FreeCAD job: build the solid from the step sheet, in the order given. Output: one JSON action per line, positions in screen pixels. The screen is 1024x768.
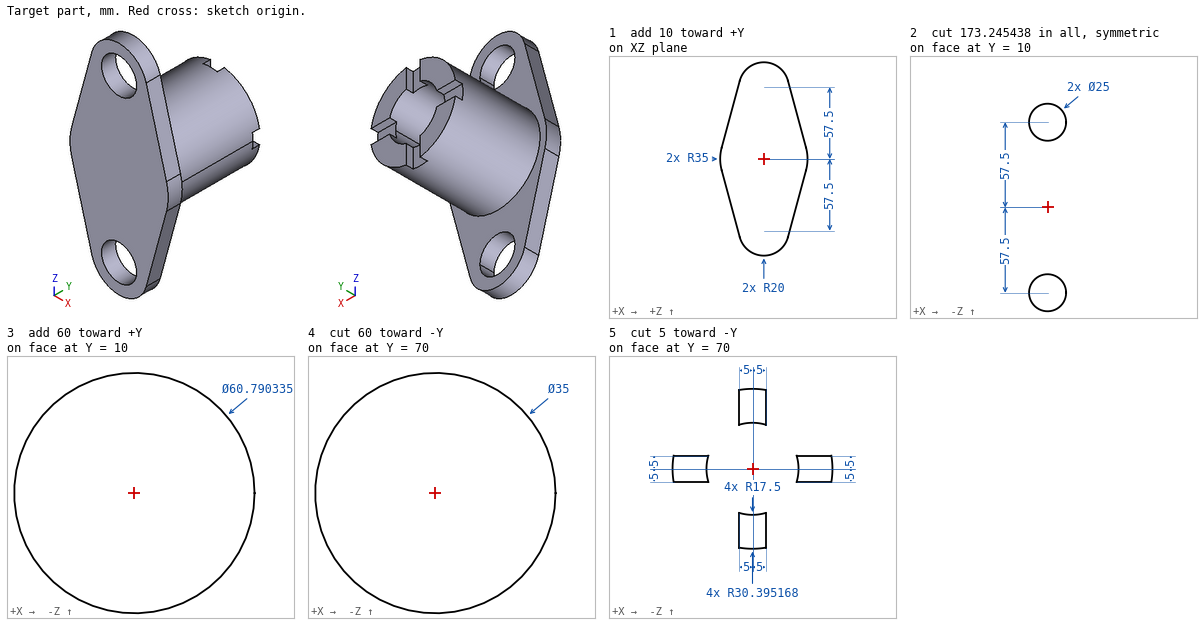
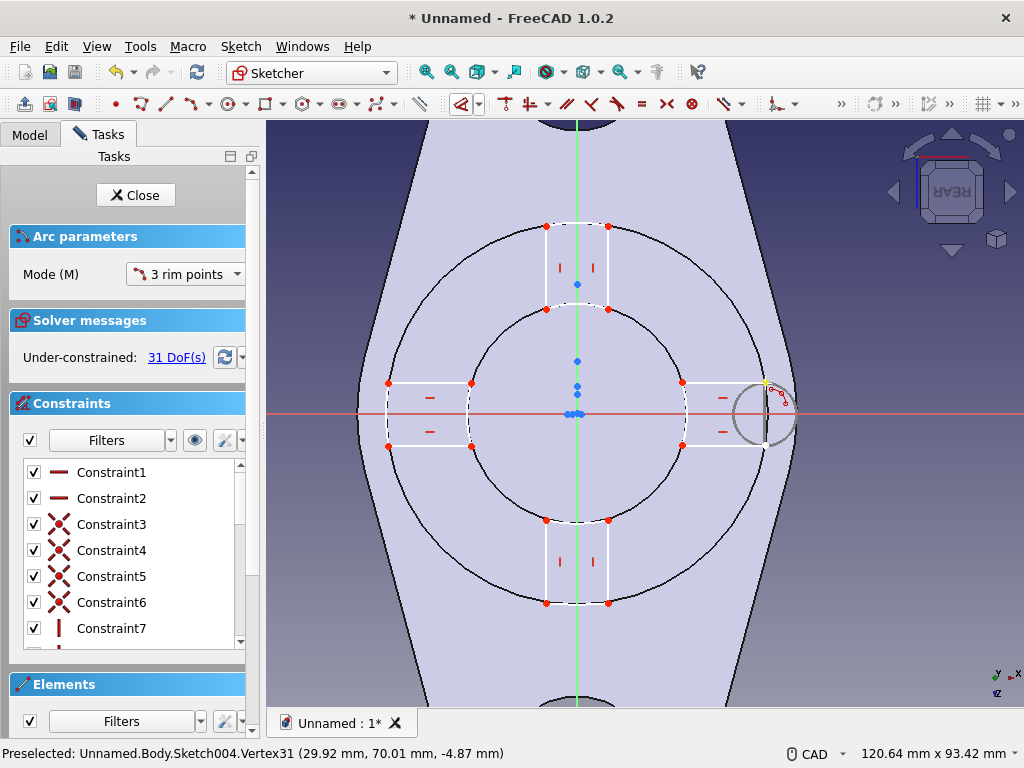
{"action": "scroll", "coordinate": [768, 420], "scroll_direction": "up", "scroll_amount": 10}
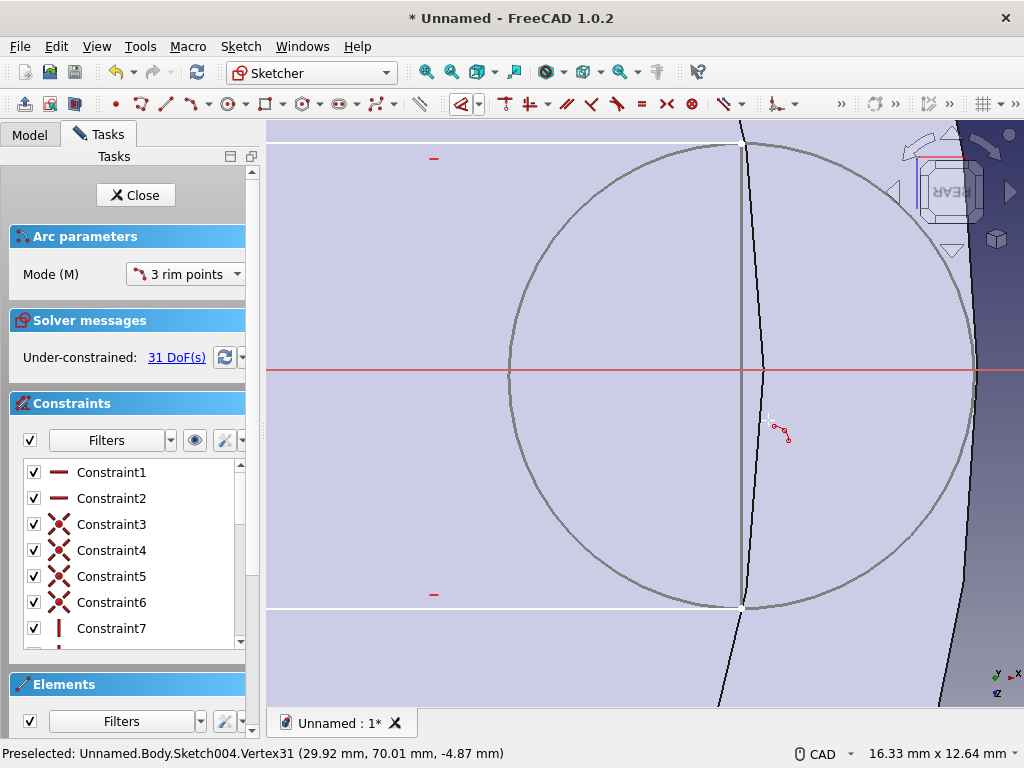
{"action": "left_click", "coordinate": [763, 416]}
{"action": "key", "text": "Escape"}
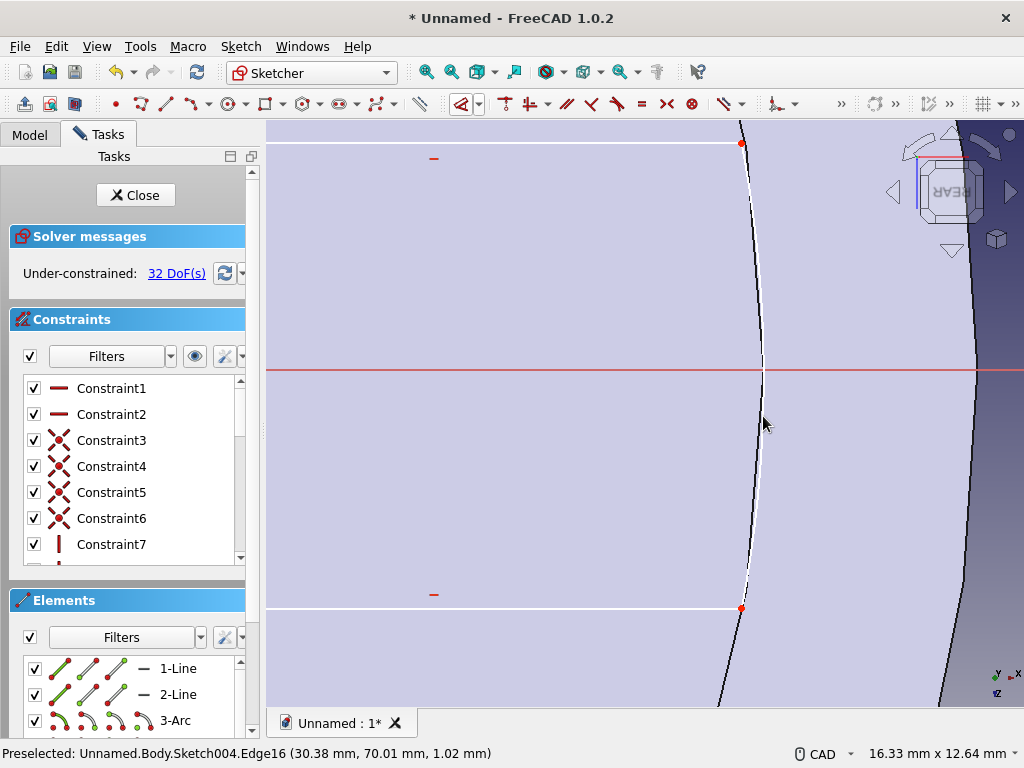
{"action": "scroll", "coordinate": [768, 420], "scroll_direction": "down", "scroll_amount": 10}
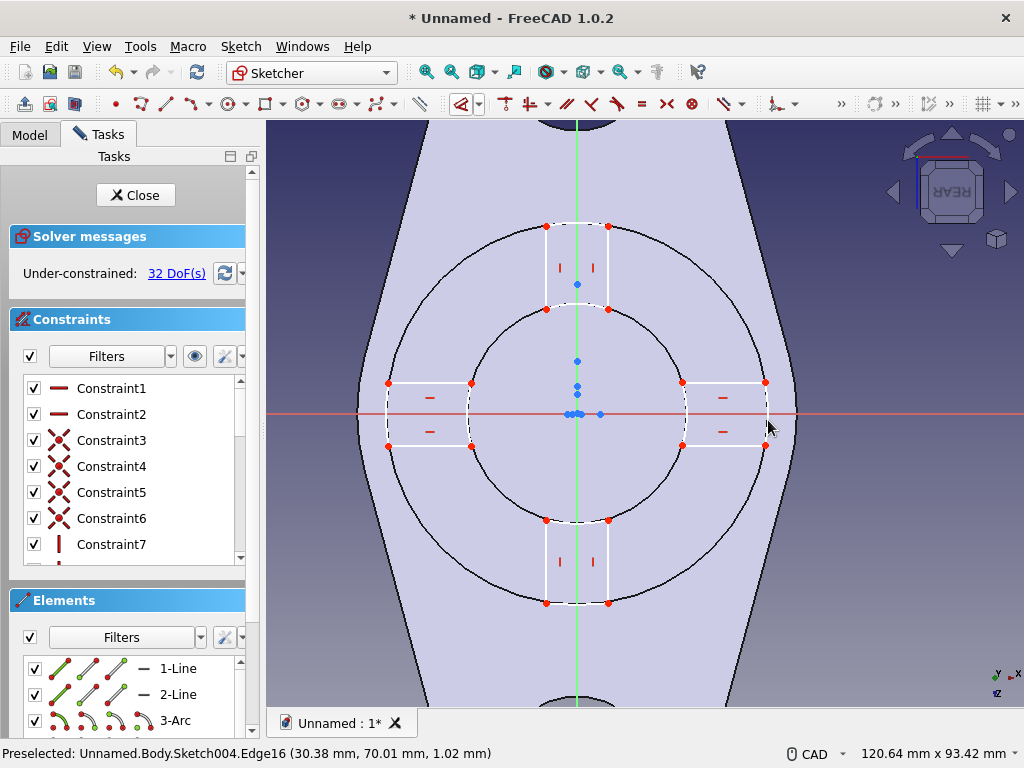
{"action": "left_click", "coordinate": [468, 402]}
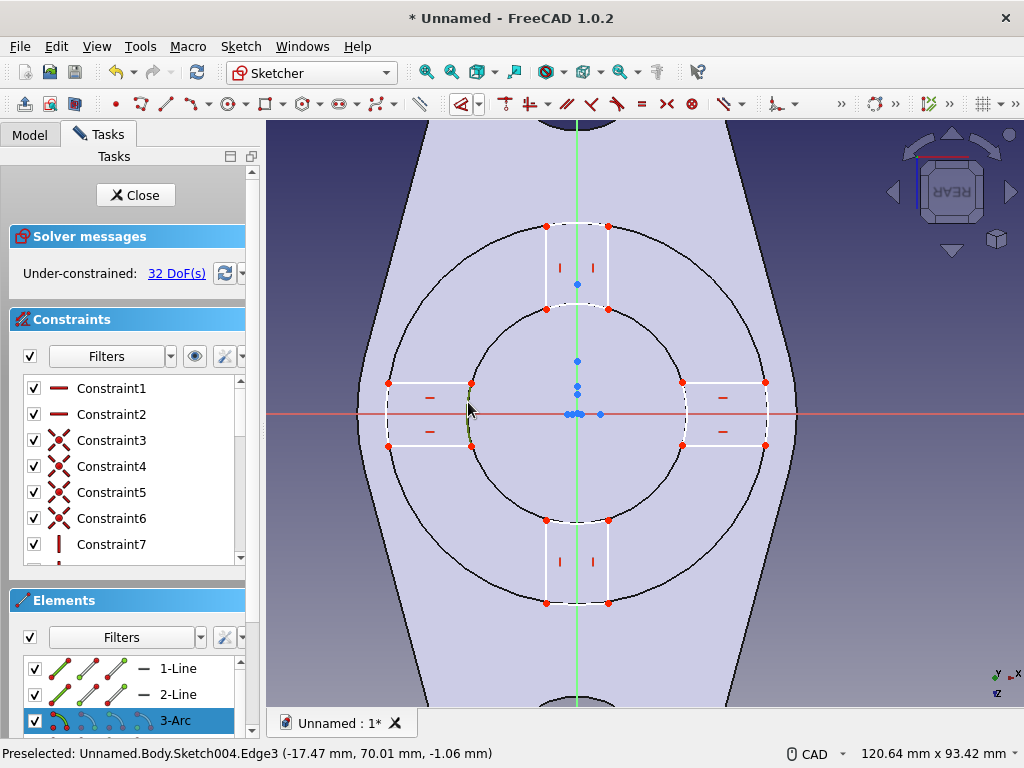
{"action": "left_click", "coordinate": [386, 402]}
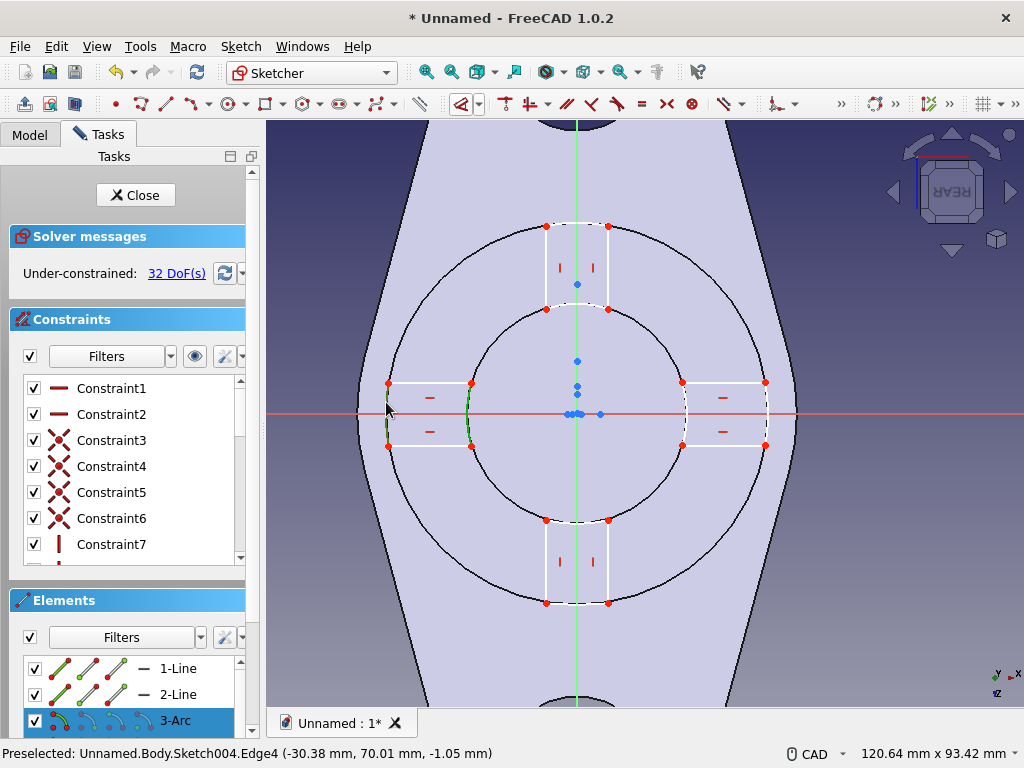
{"action": "key", "text": "c"}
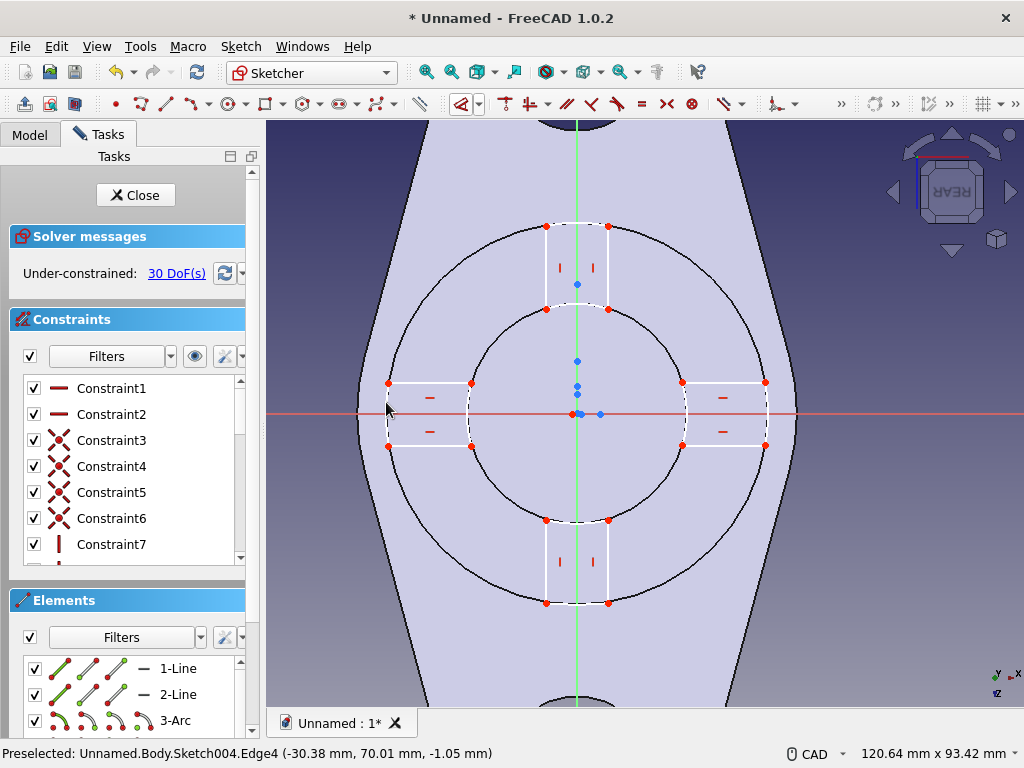
{"action": "left_click", "coordinate": [468, 402]}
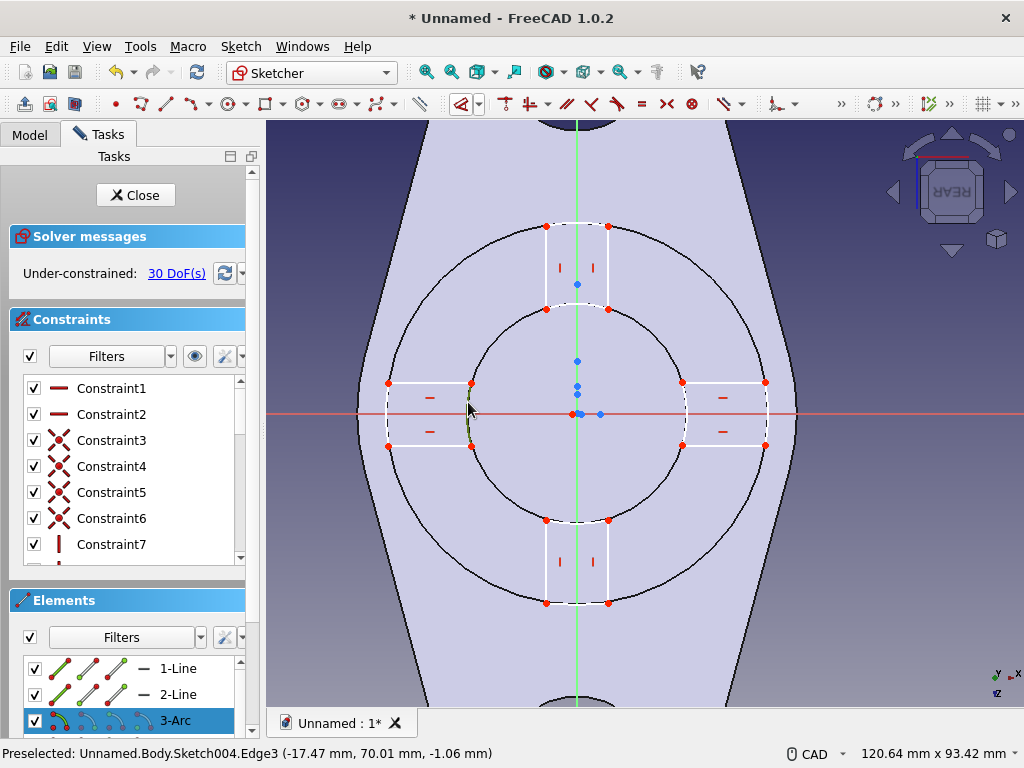
{"action": "left_click", "coordinate": [565, 604]}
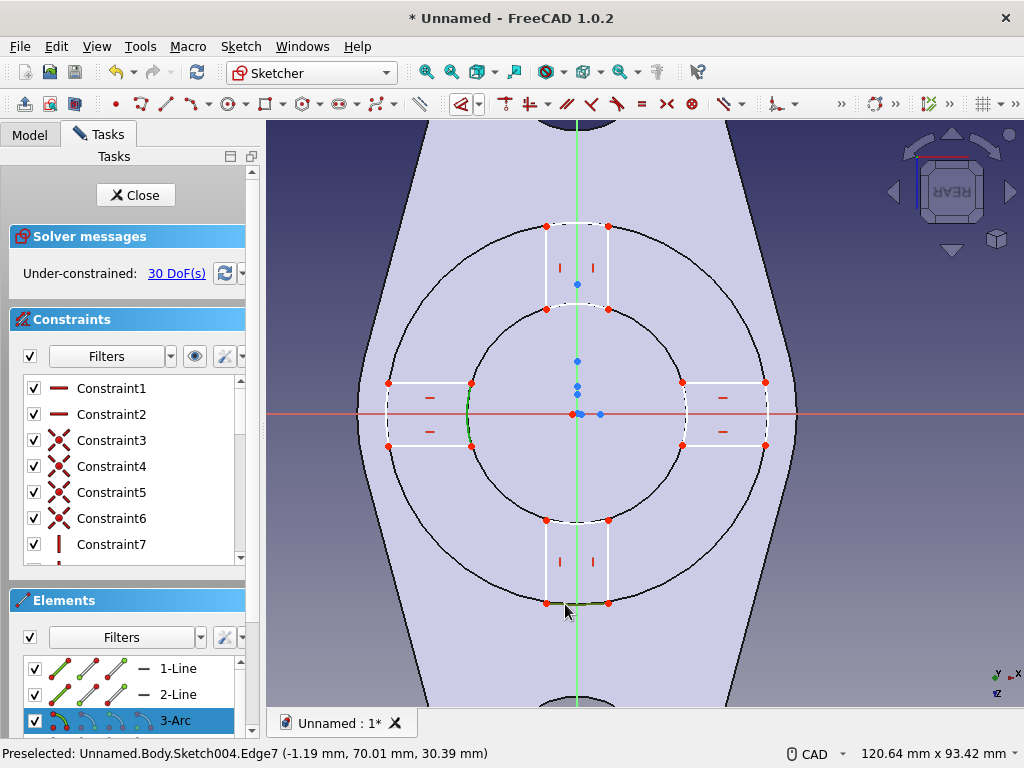
{"action": "left_click", "coordinate": [505, 104]}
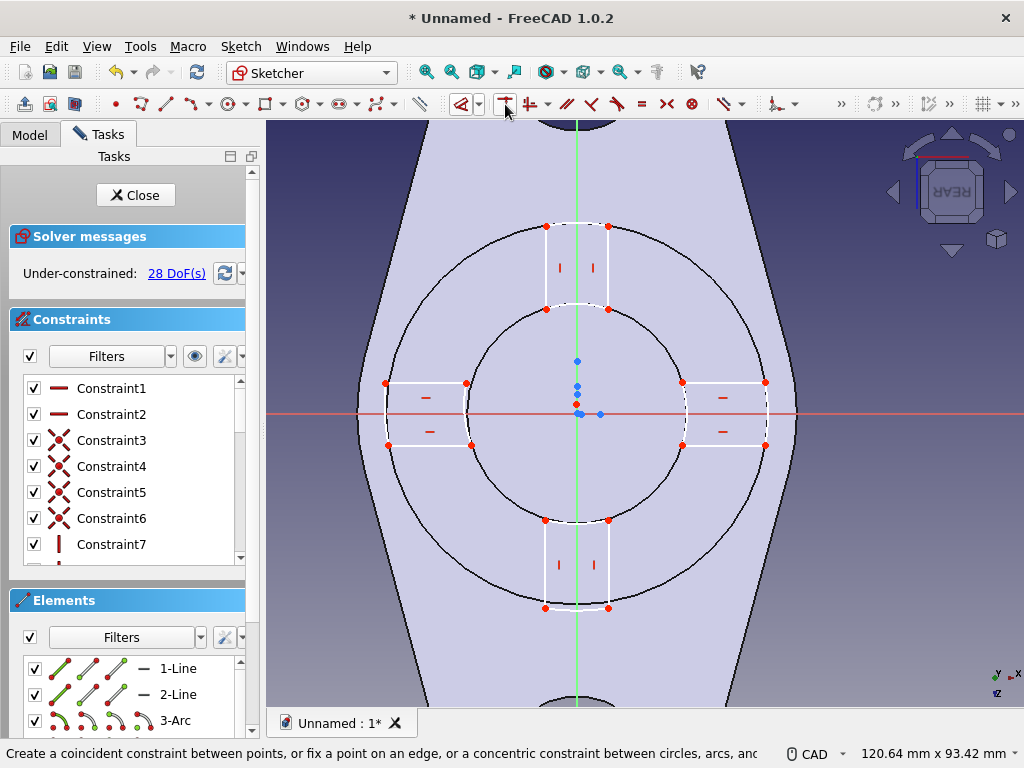
{"action": "left_click", "coordinate": [464, 402]}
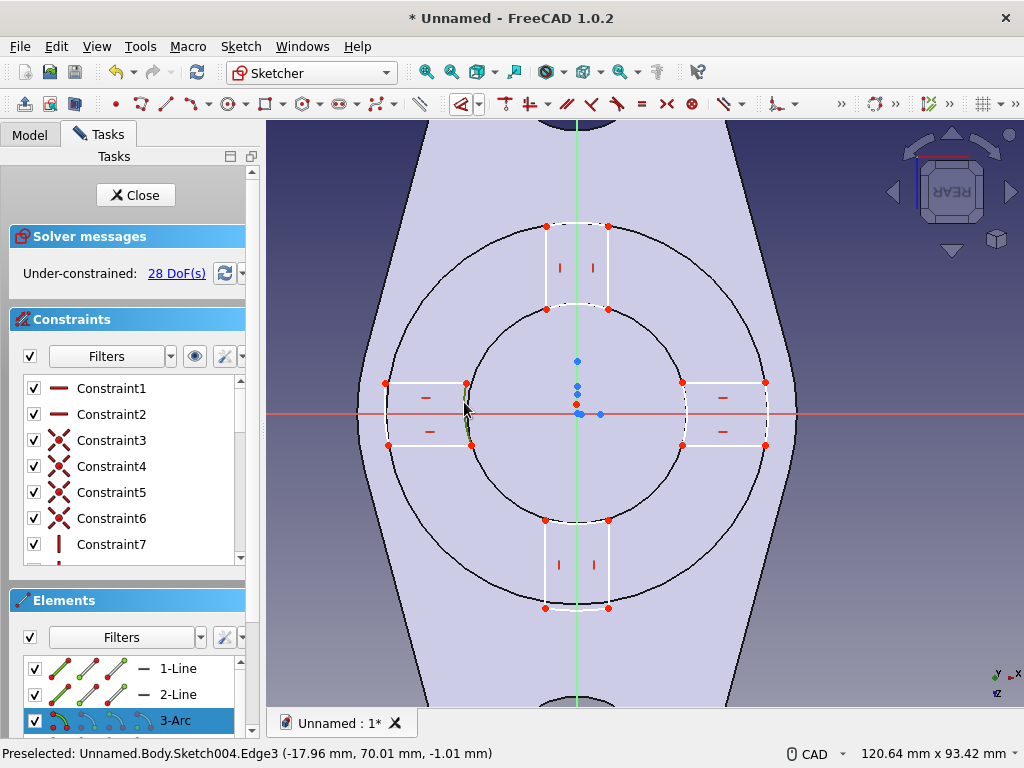
{"action": "left_click", "coordinate": [564, 523]}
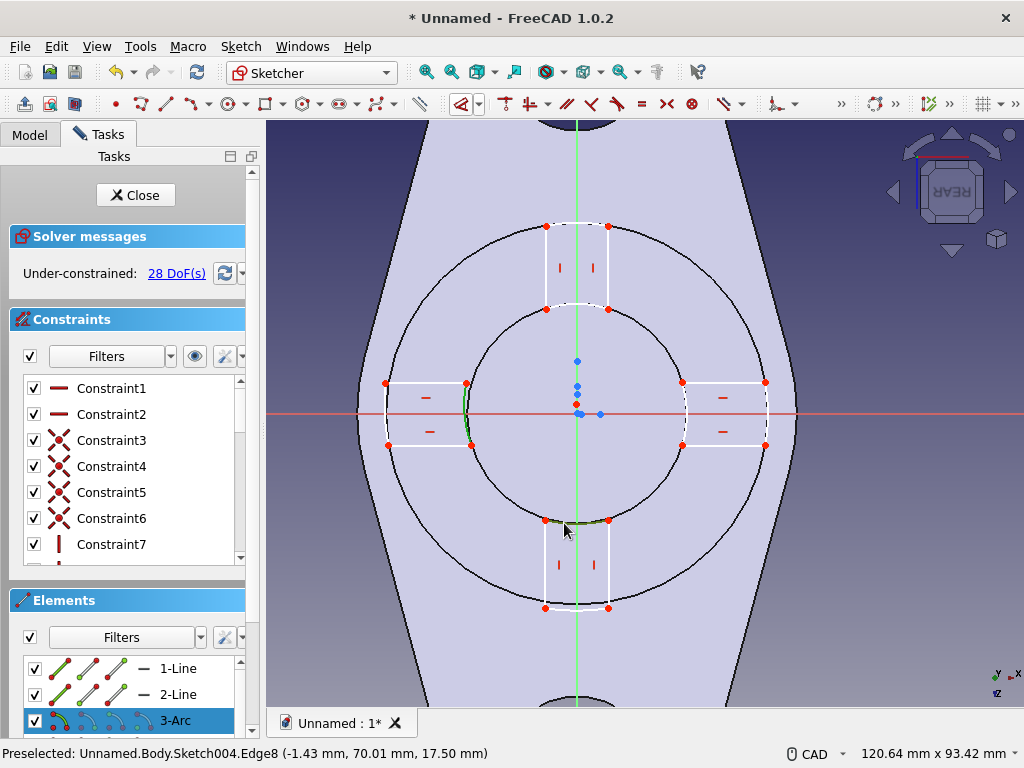
{"action": "left_click", "coordinate": [505, 104]}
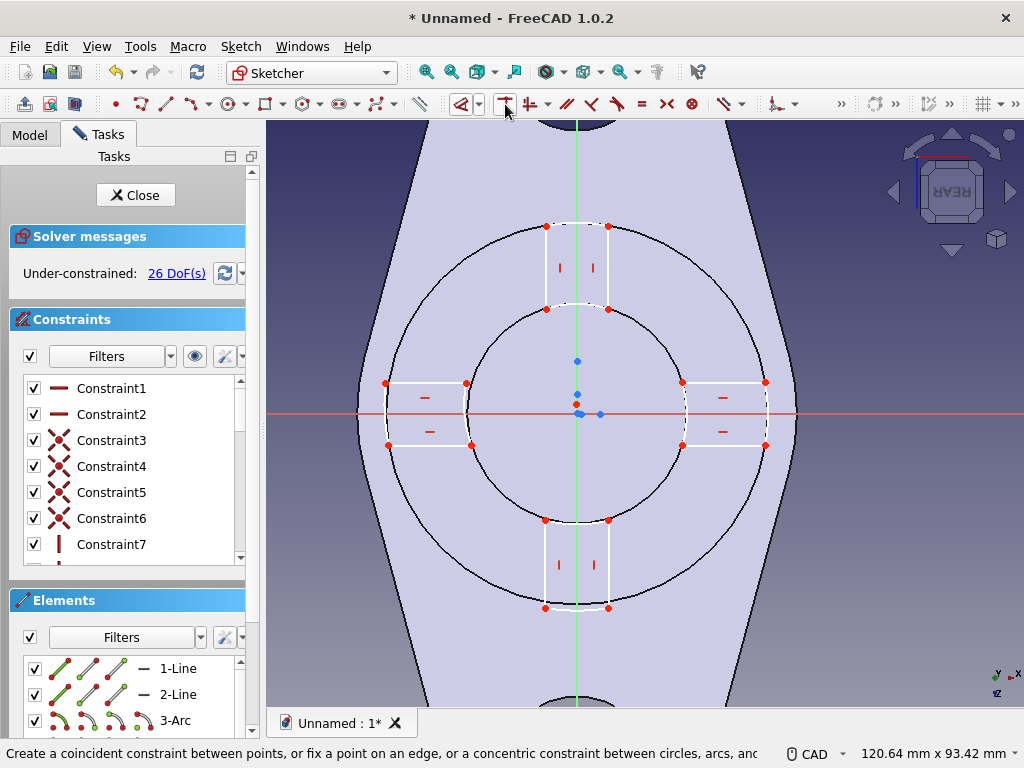
{"action": "left_click", "coordinate": [464, 402]}